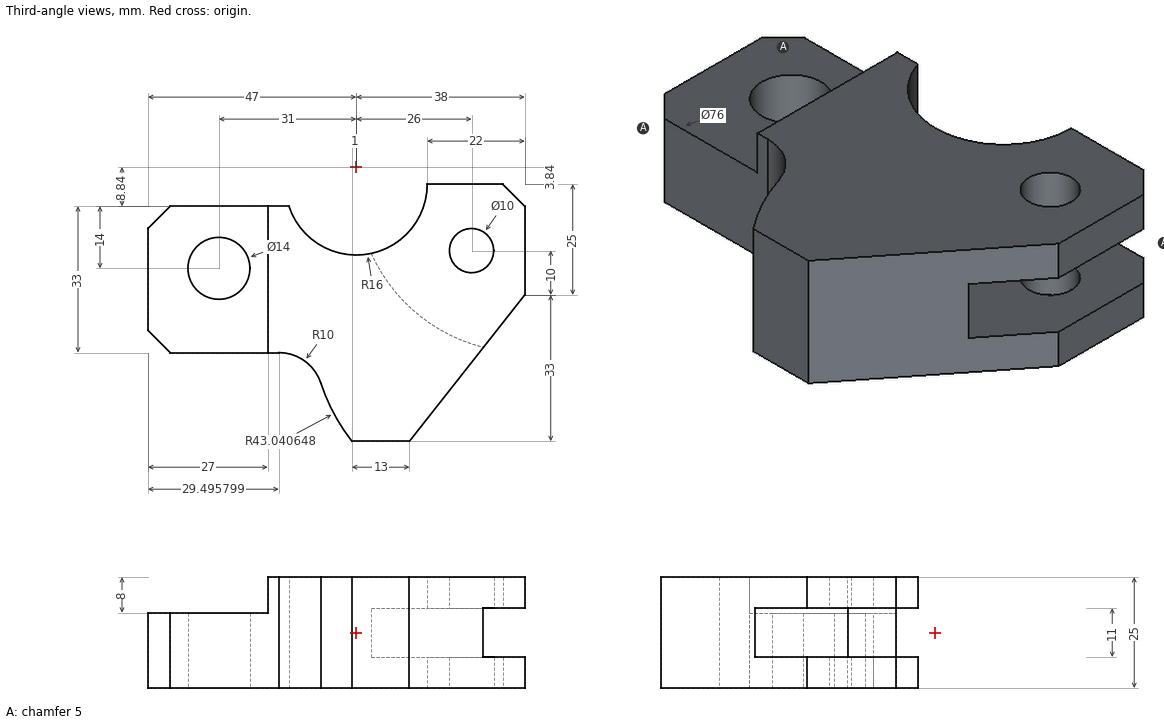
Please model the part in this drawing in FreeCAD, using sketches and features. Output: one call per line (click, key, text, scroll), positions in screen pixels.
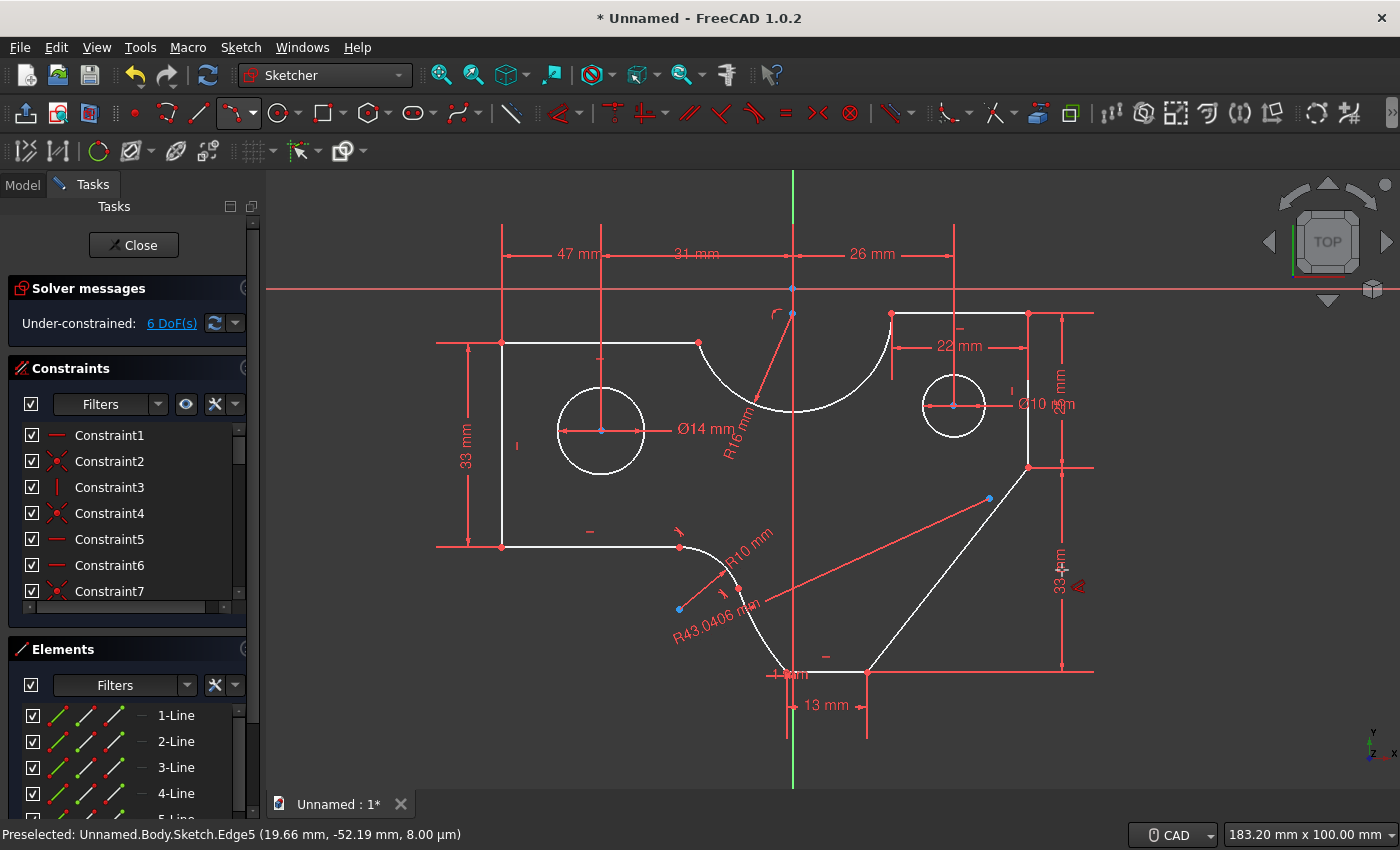
click(698, 343)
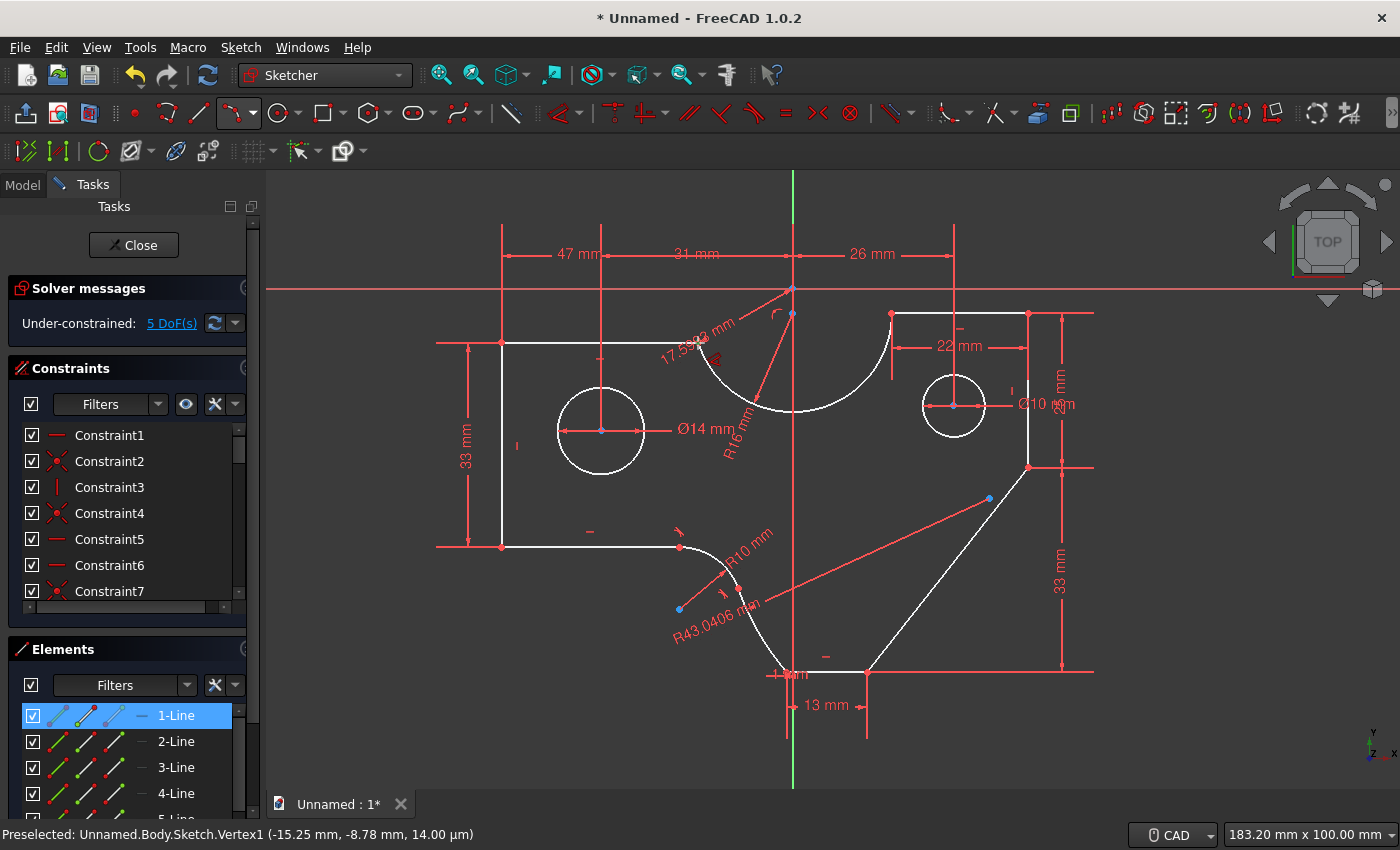
click(601, 431)
click(567, 367)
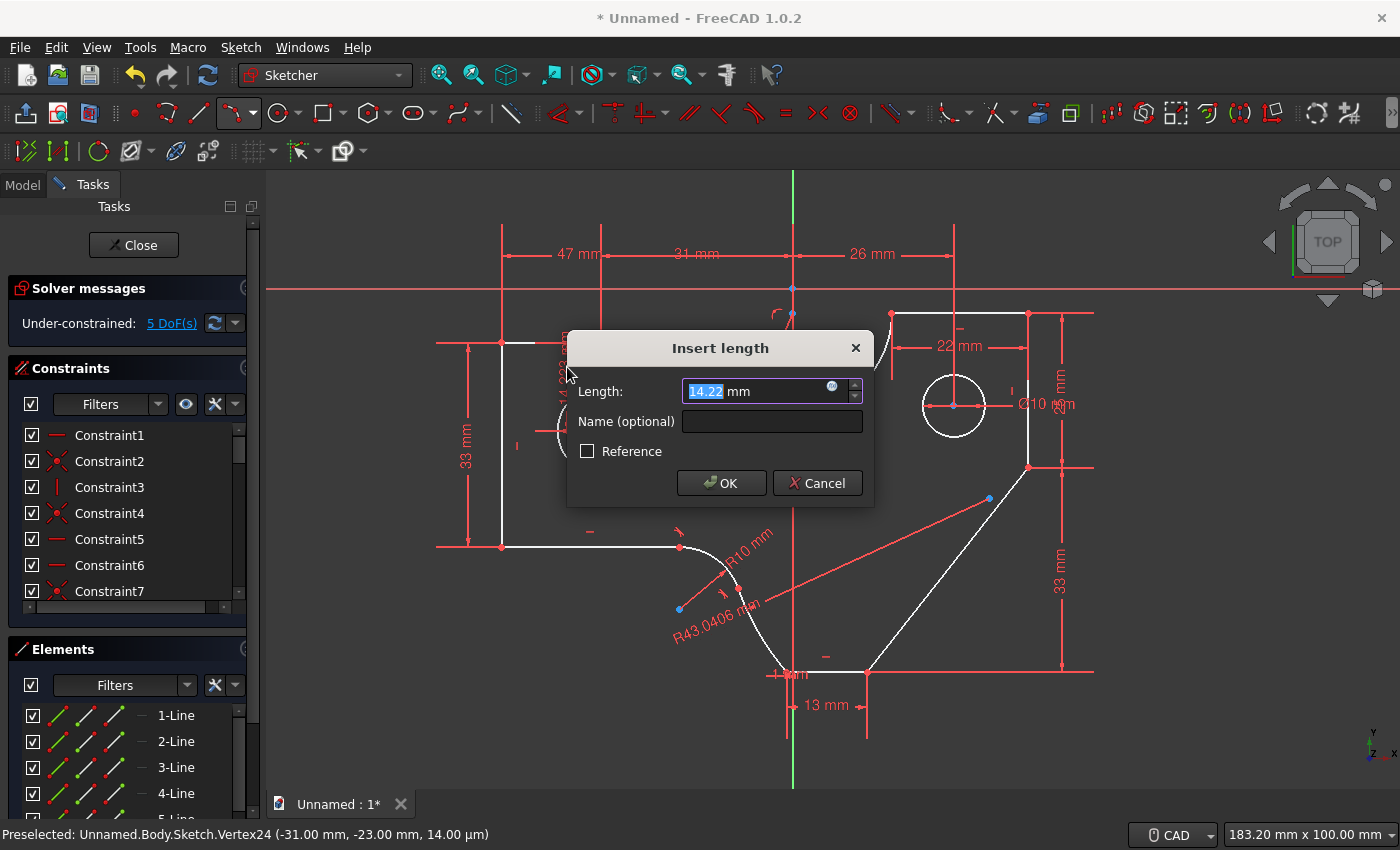
text(14)
key(Return)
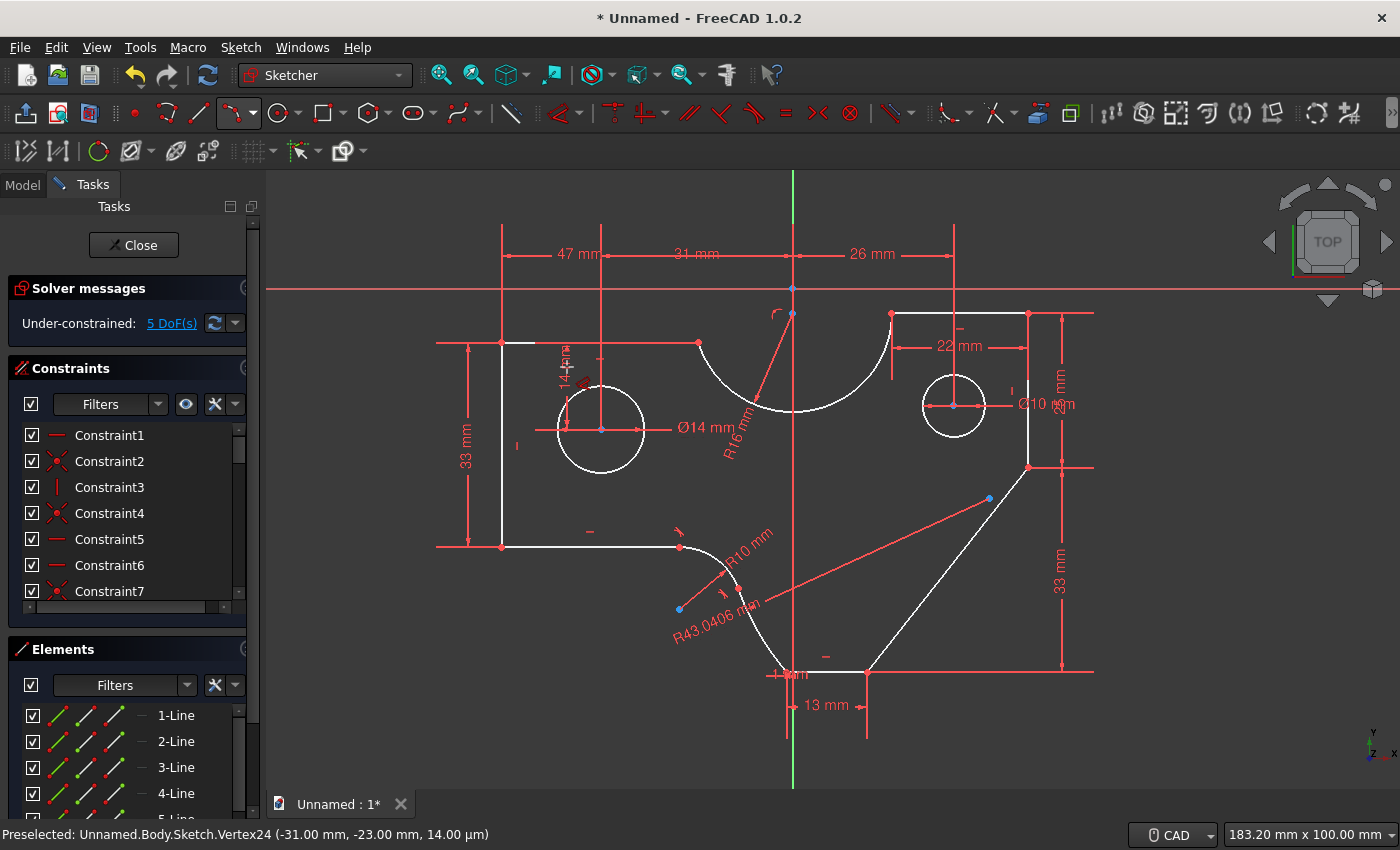
click(1028, 468)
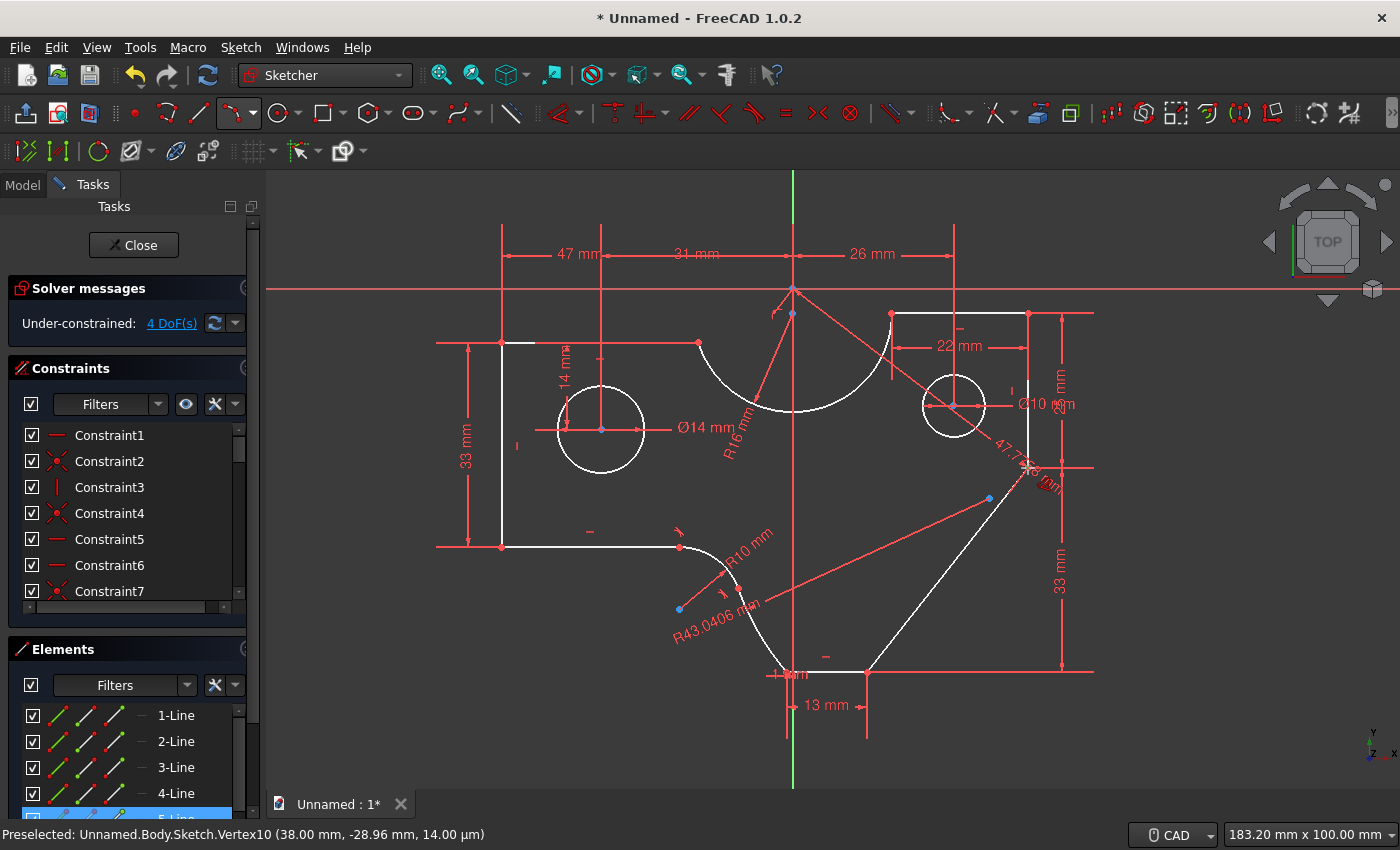
click(954, 406)
click(1062, 437)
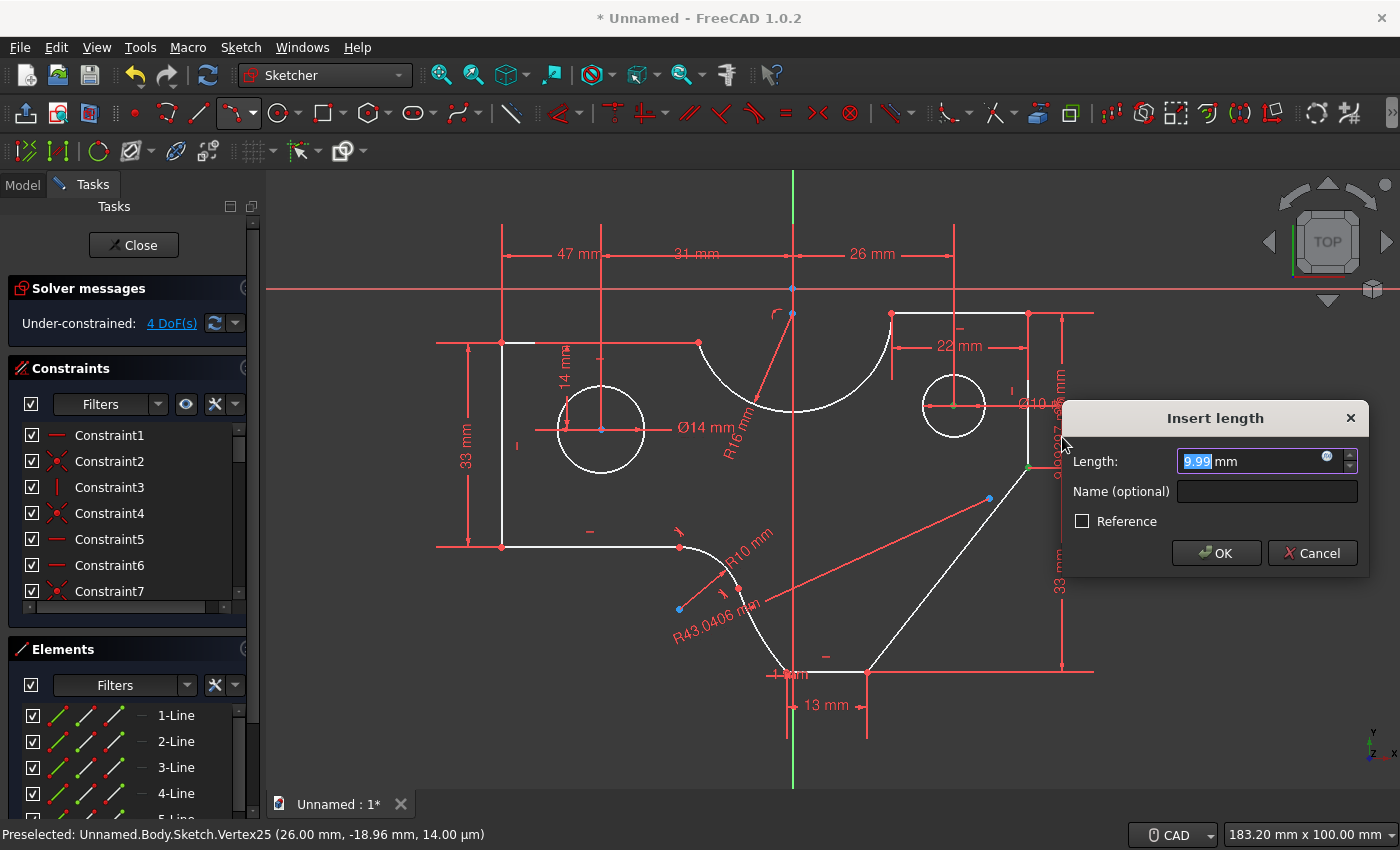
text(10)
key(Return)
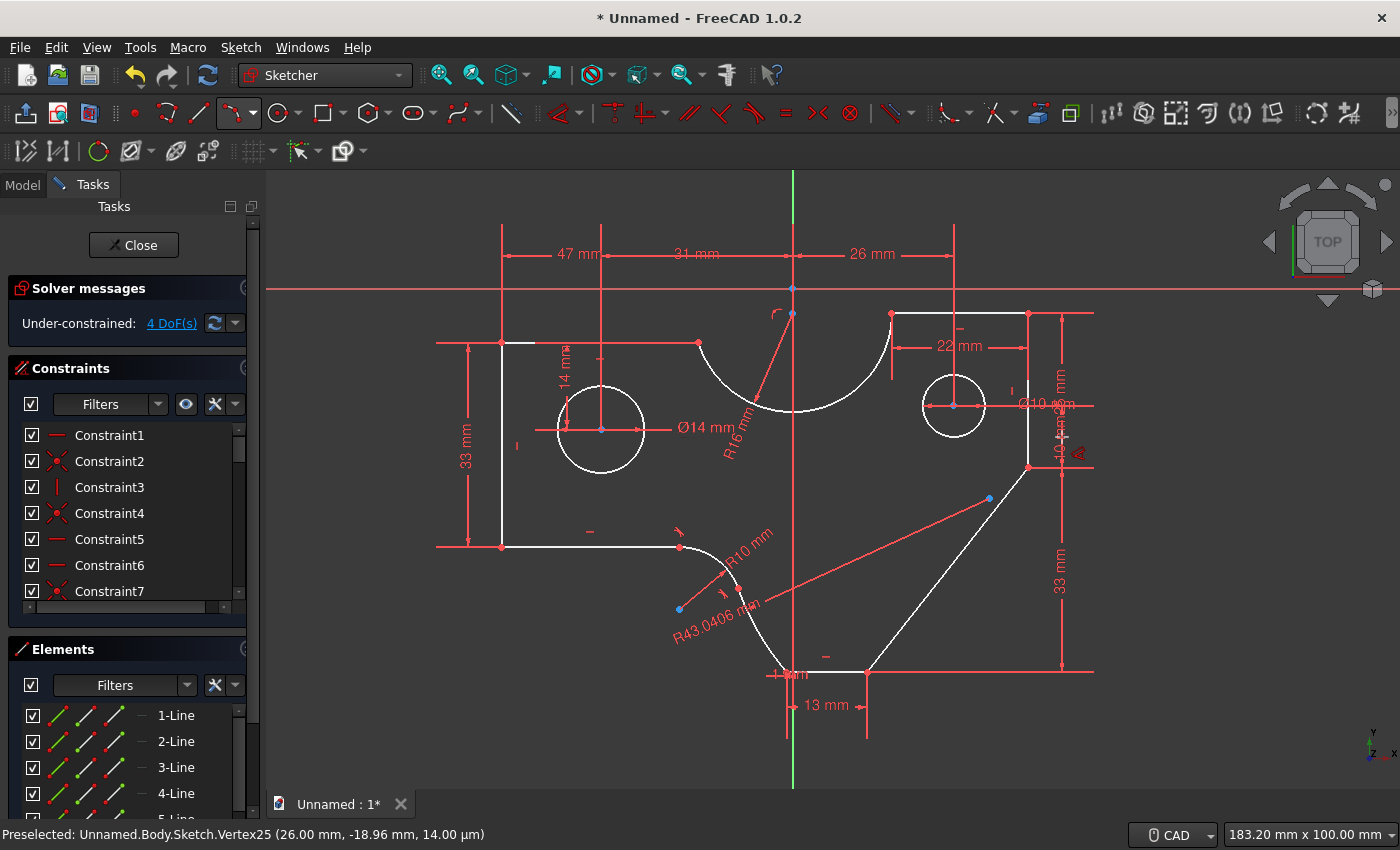
click(698, 343)
click(664, 316)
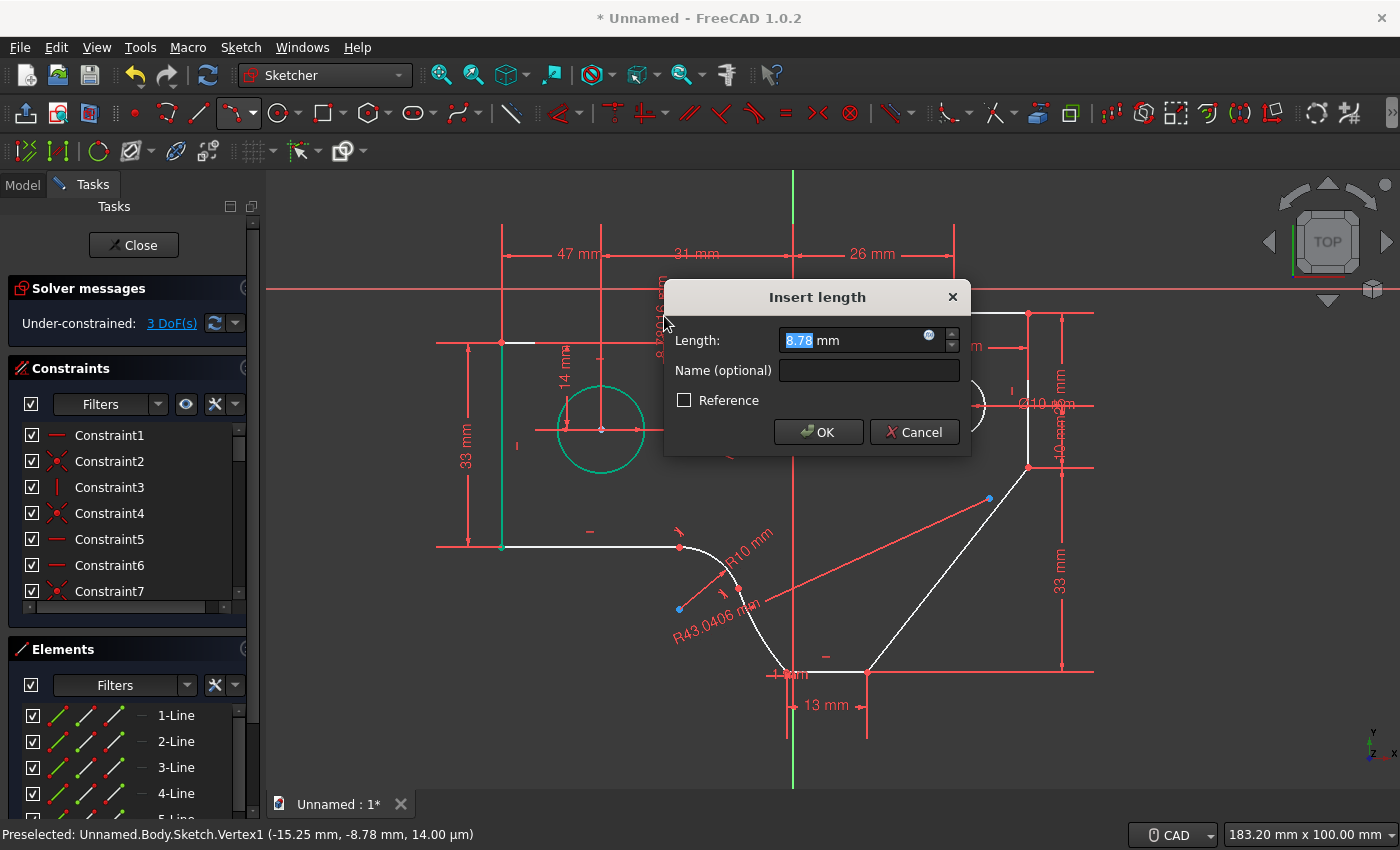
text(8.84)
key(Return)